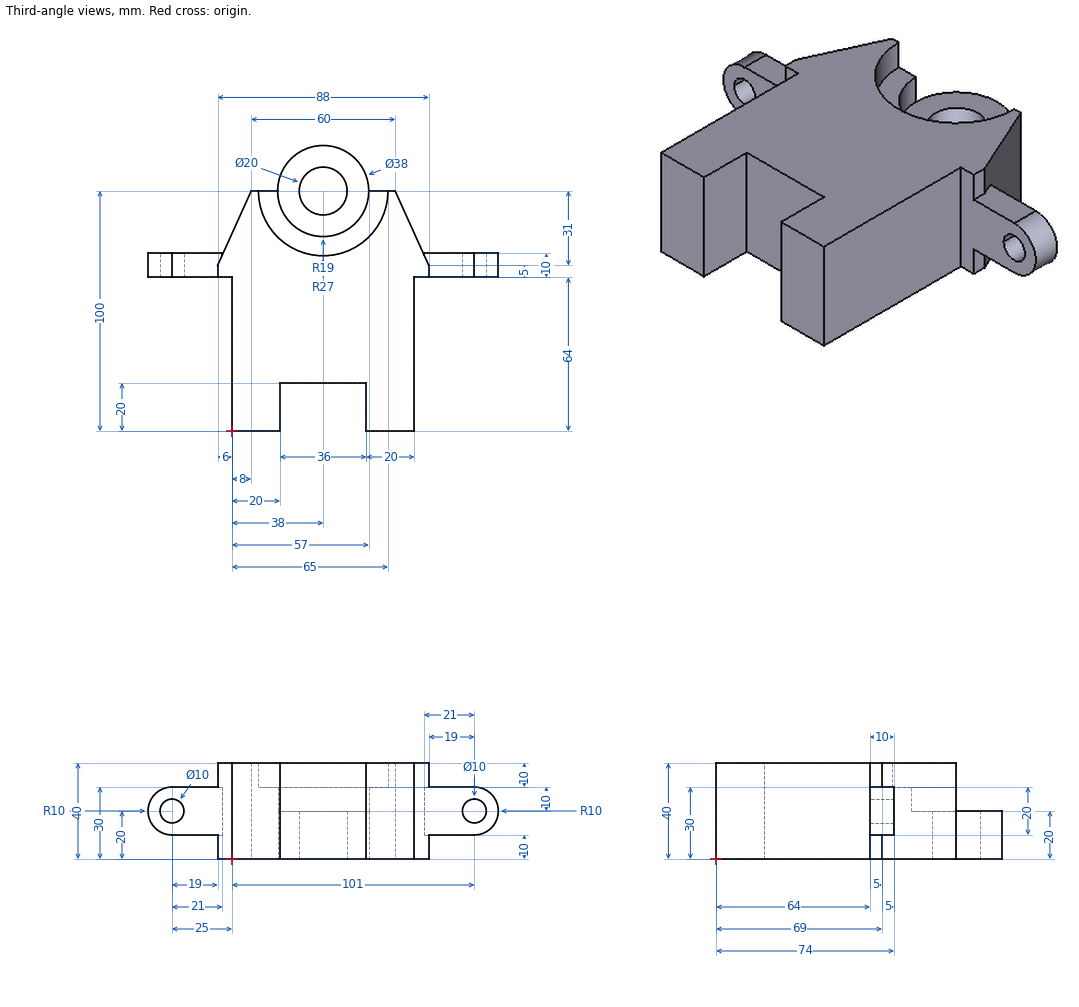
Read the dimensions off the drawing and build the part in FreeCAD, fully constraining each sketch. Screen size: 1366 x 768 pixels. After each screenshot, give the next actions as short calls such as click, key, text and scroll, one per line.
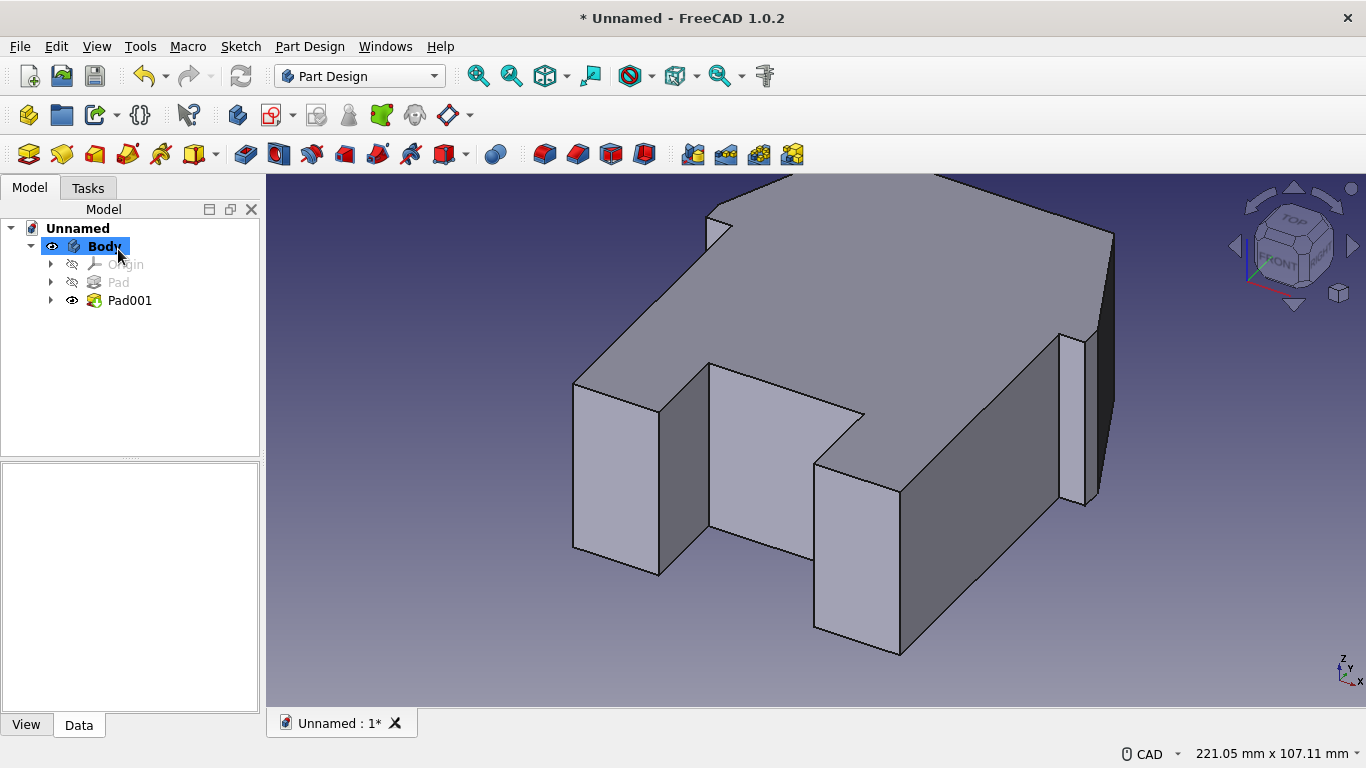
click(479, 76)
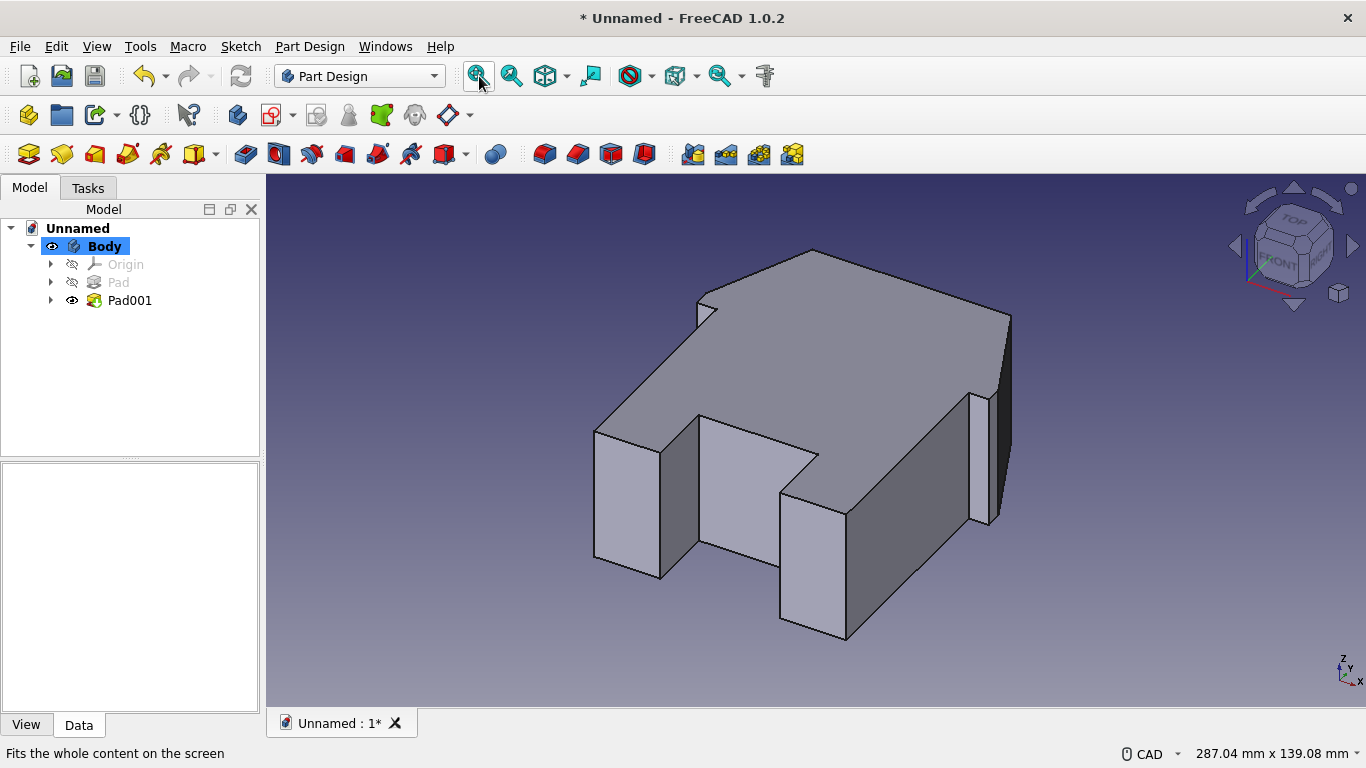
key(6)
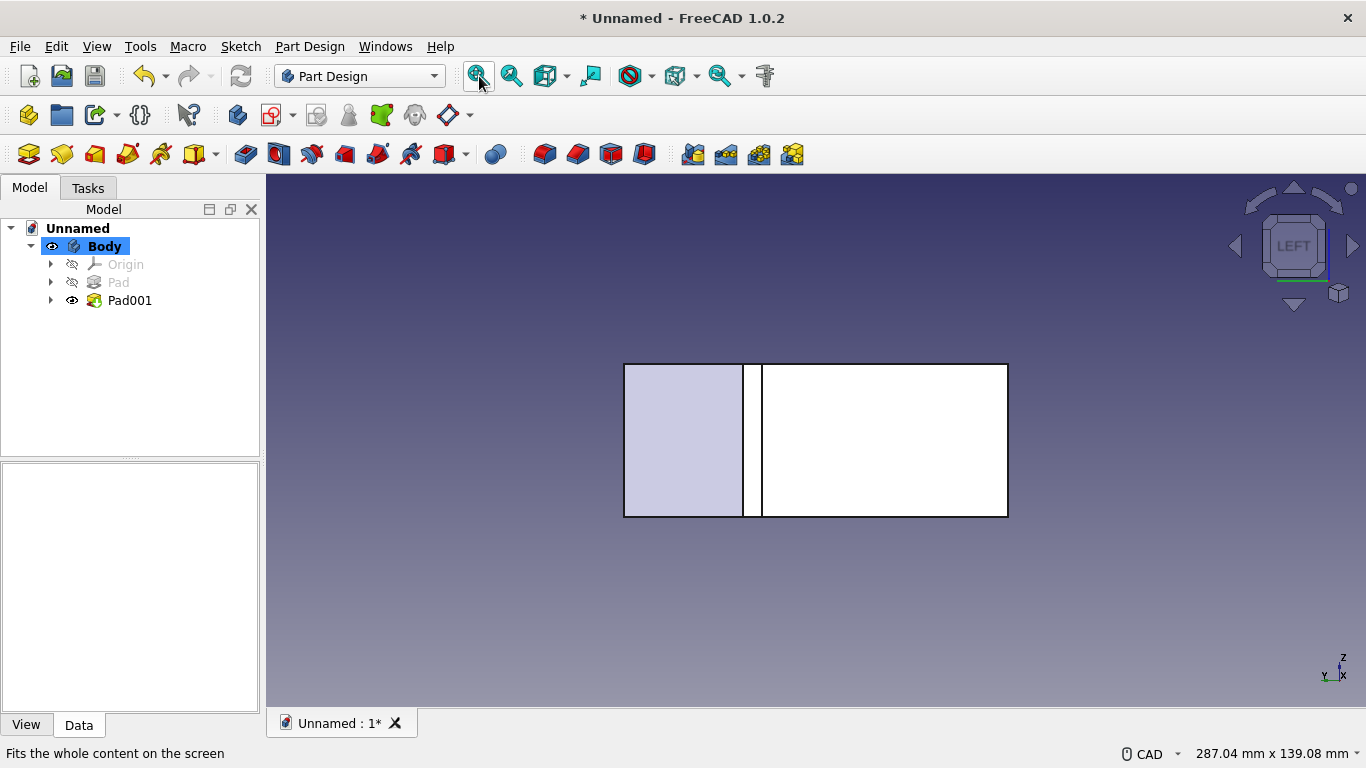
click(479, 76)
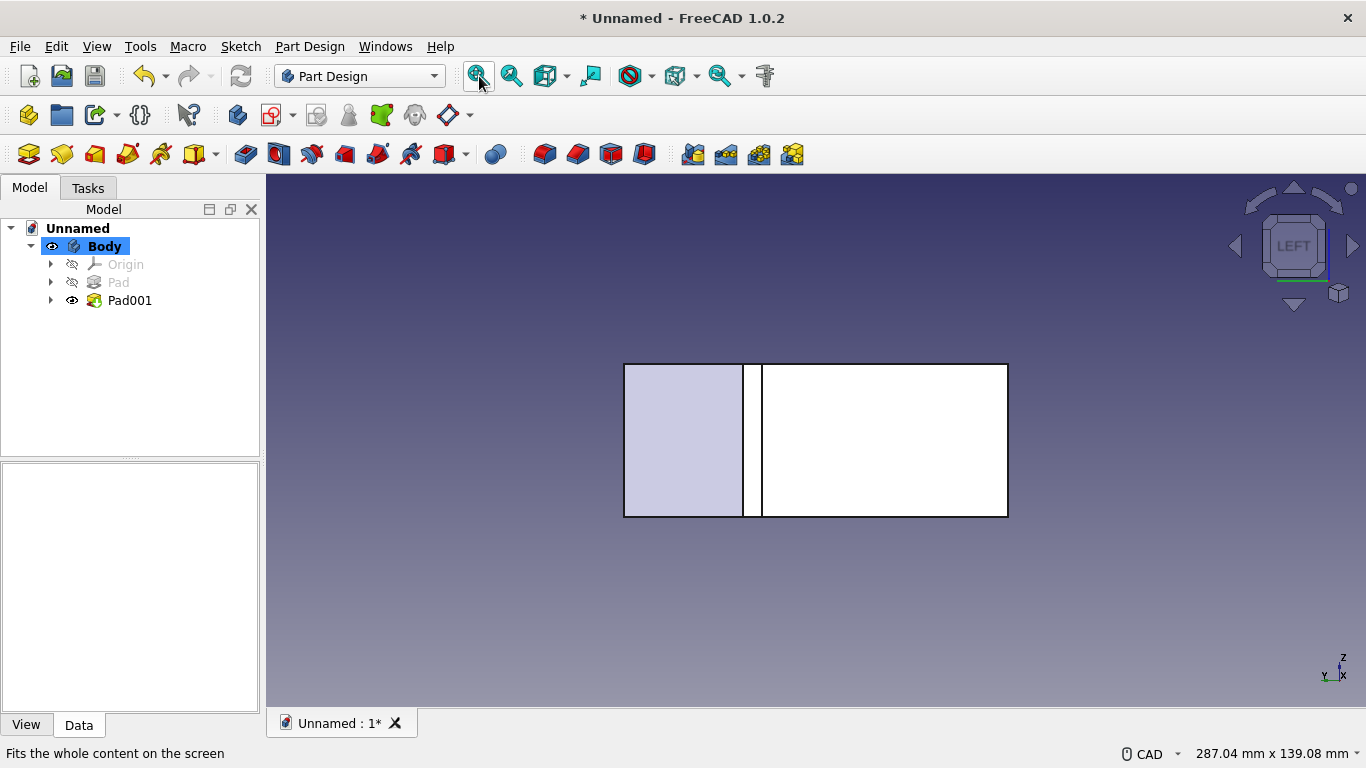
click(753, 374)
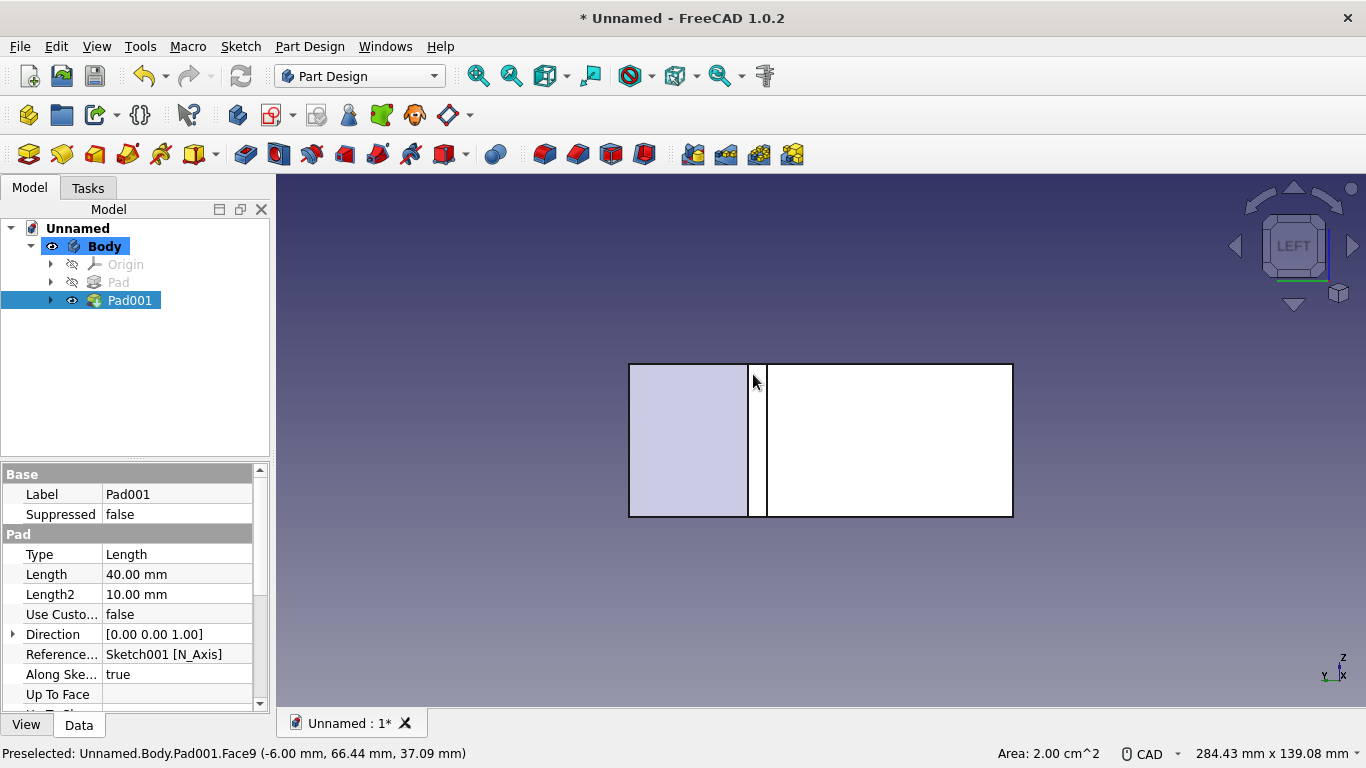
click(270, 116)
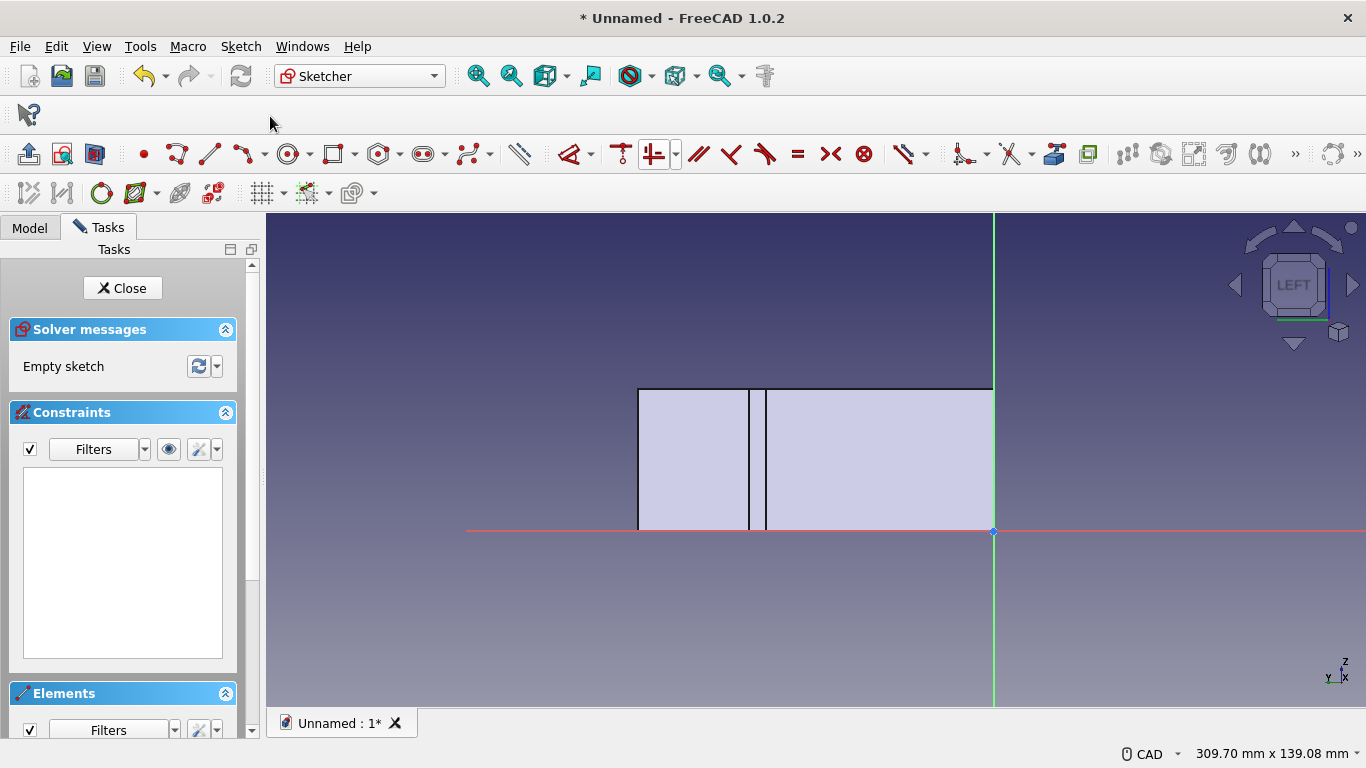
scroll(761, 460, up, 7)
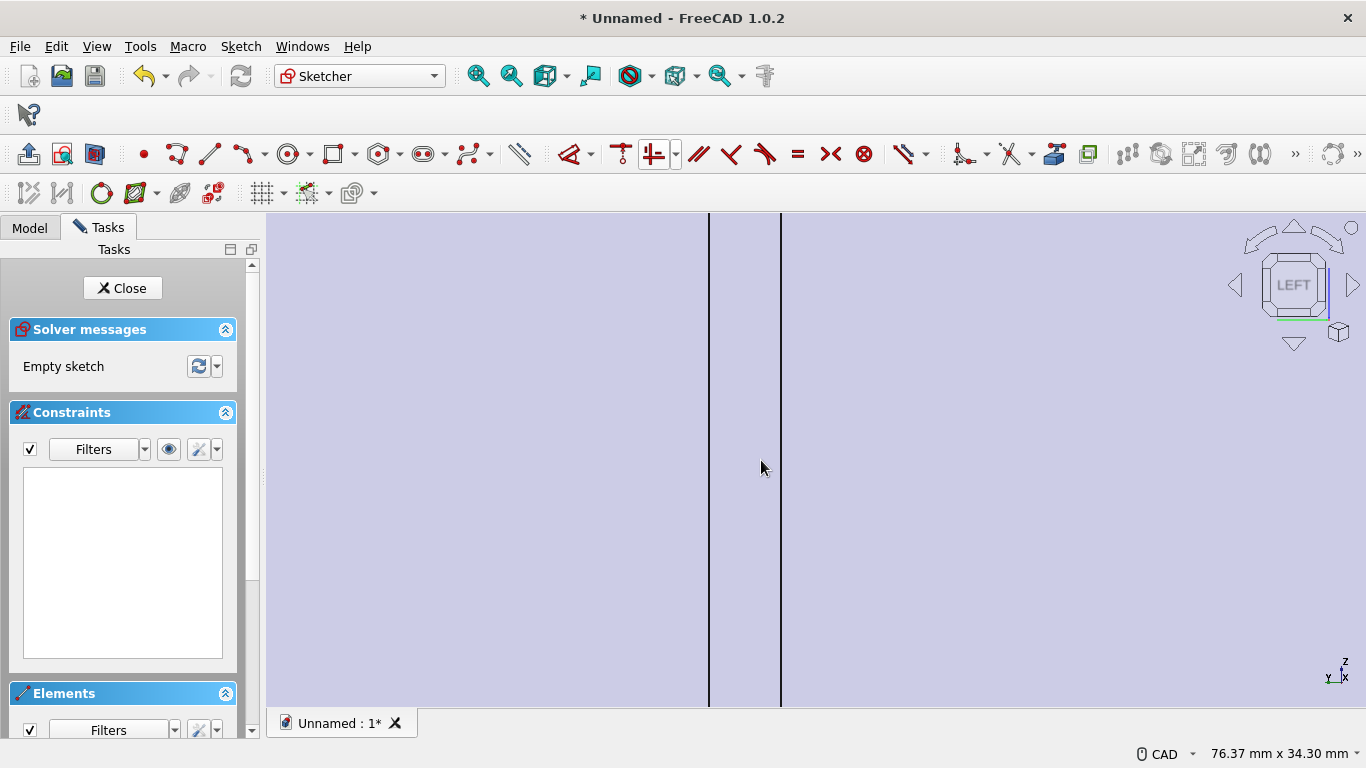
click(332, 154)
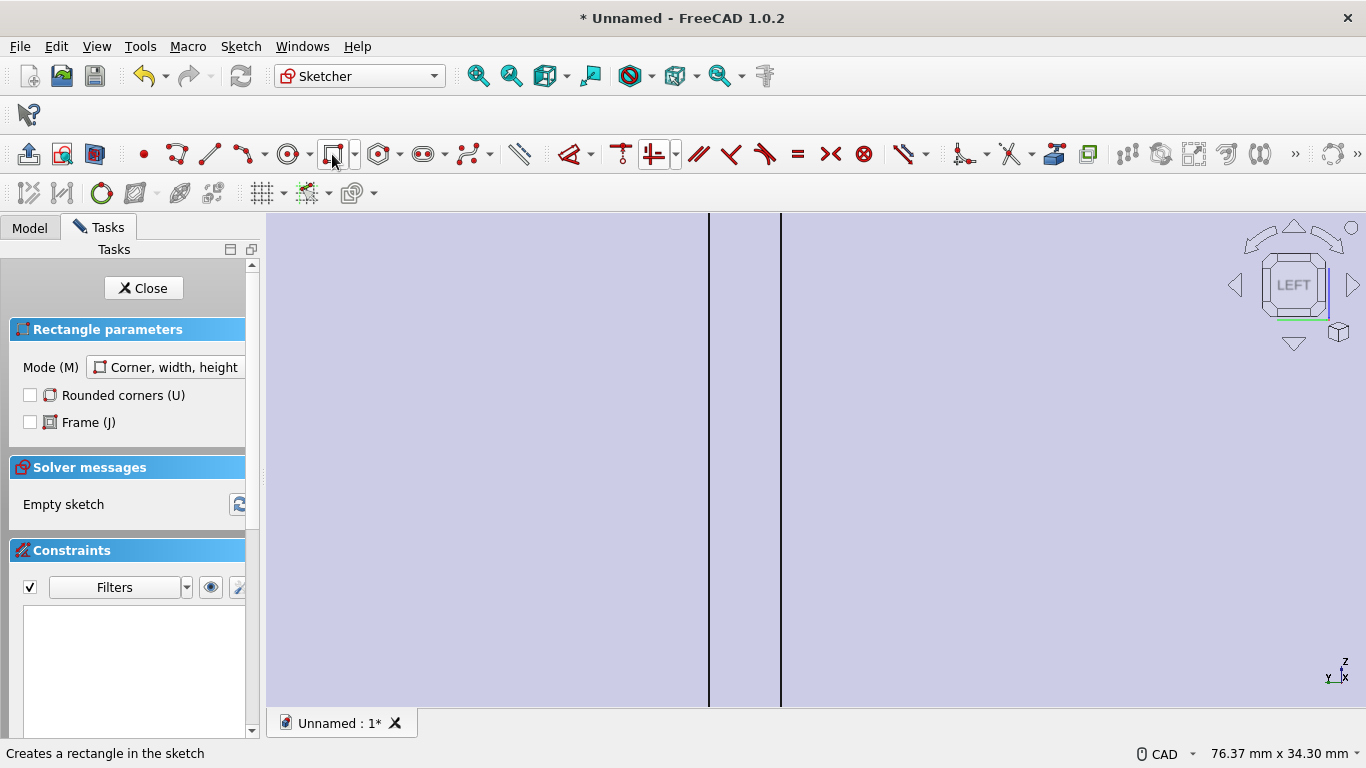
click(709, 314)
click(781, 603)
key(Escape)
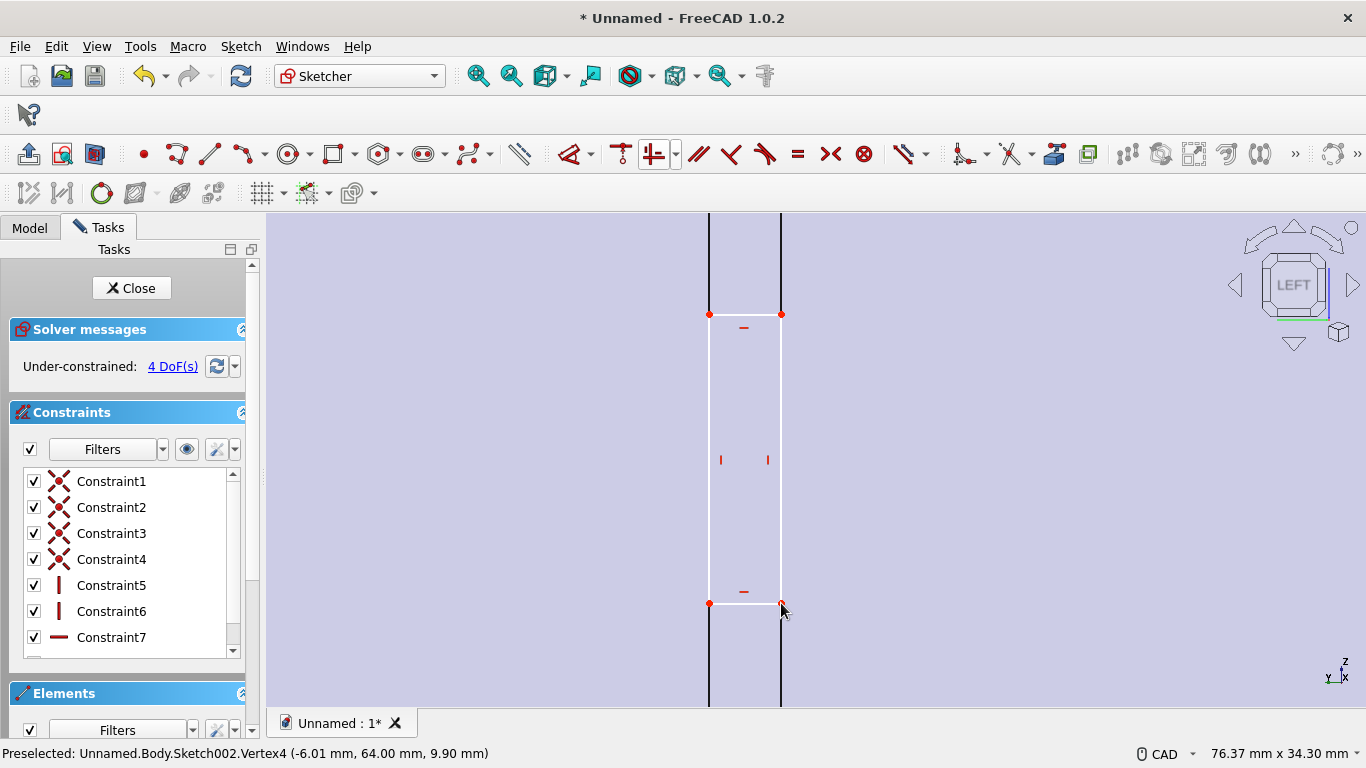
click(568, 154)